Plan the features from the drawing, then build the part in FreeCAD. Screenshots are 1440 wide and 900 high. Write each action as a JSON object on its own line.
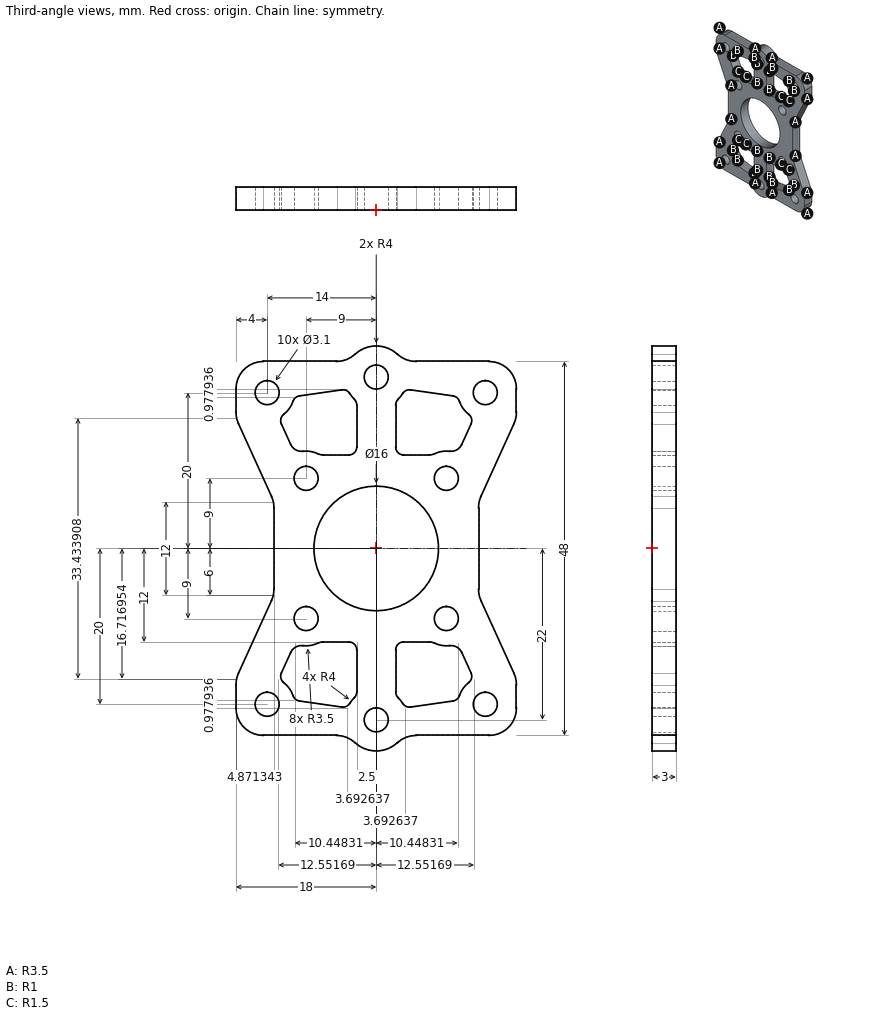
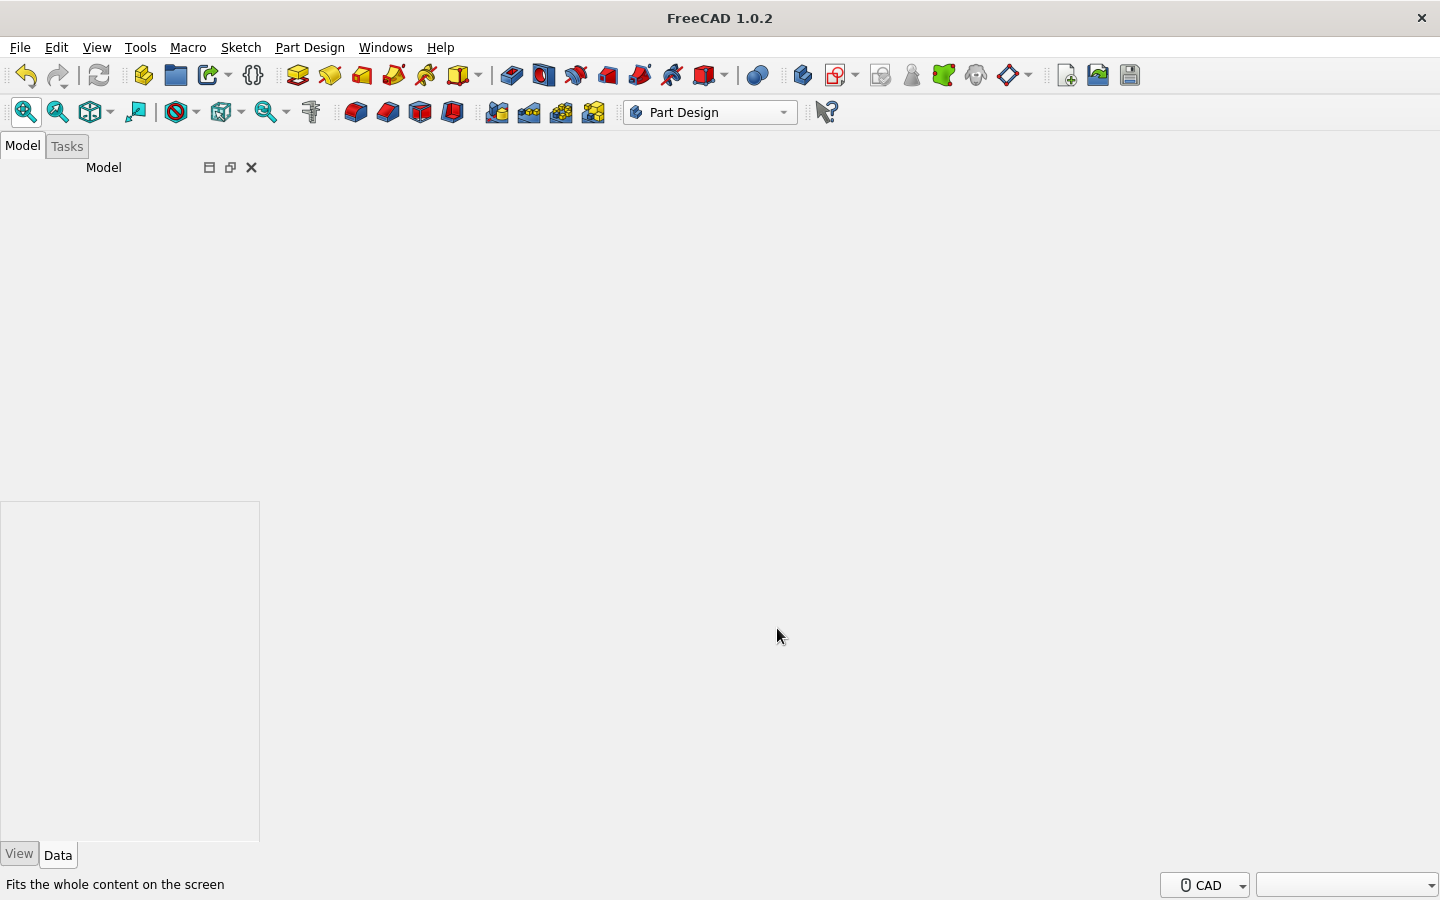
{"action": "left_click", "coordinate": [1066, 76]}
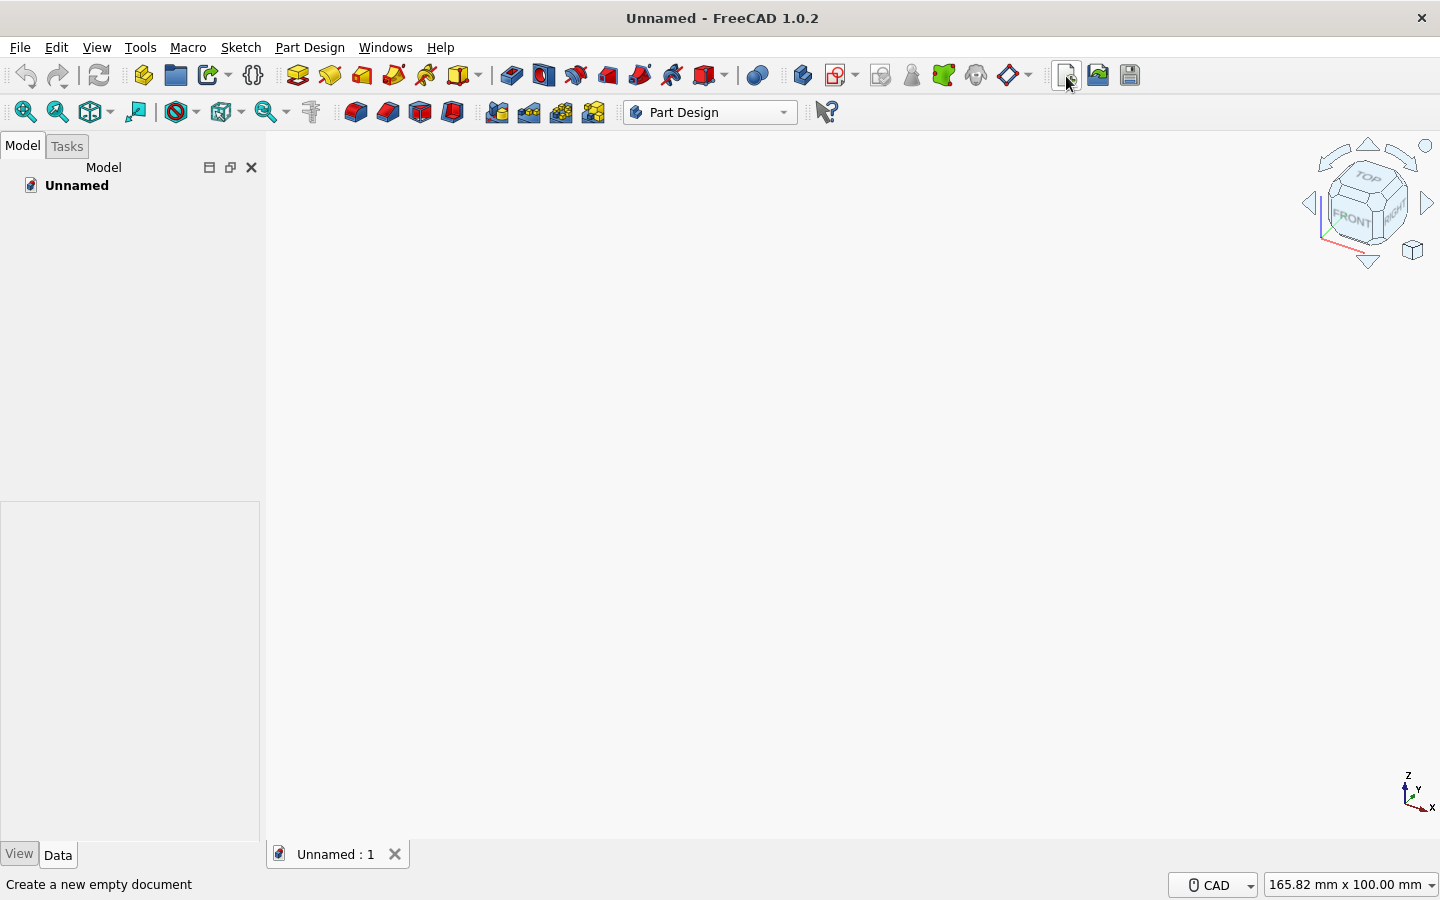
{"action": "left_click", "coordinate": [836, 76]}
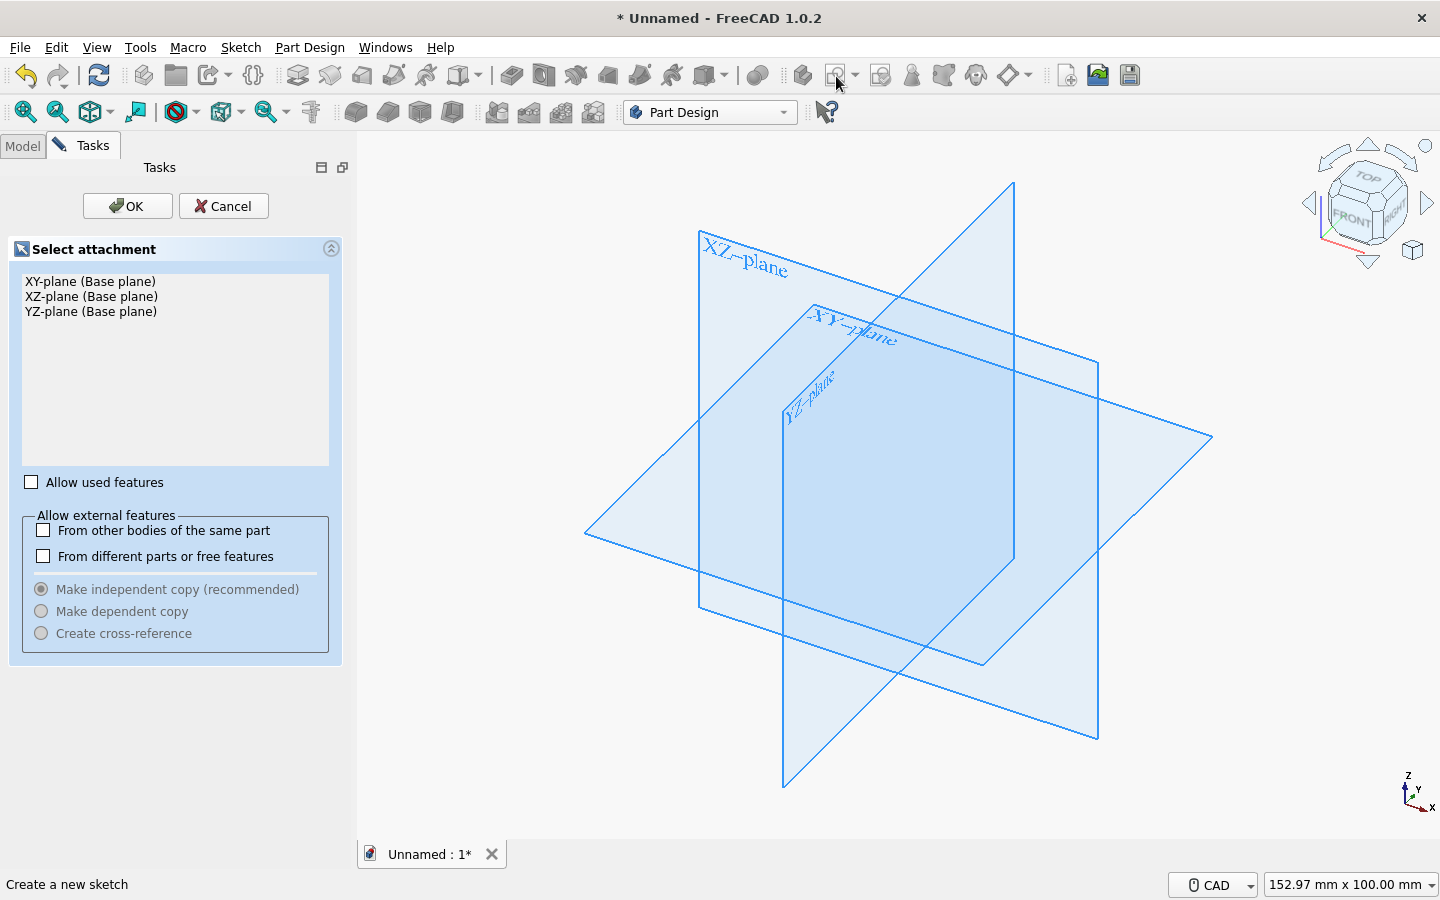
{"action": "left_click", "coordinate": [82, 296]}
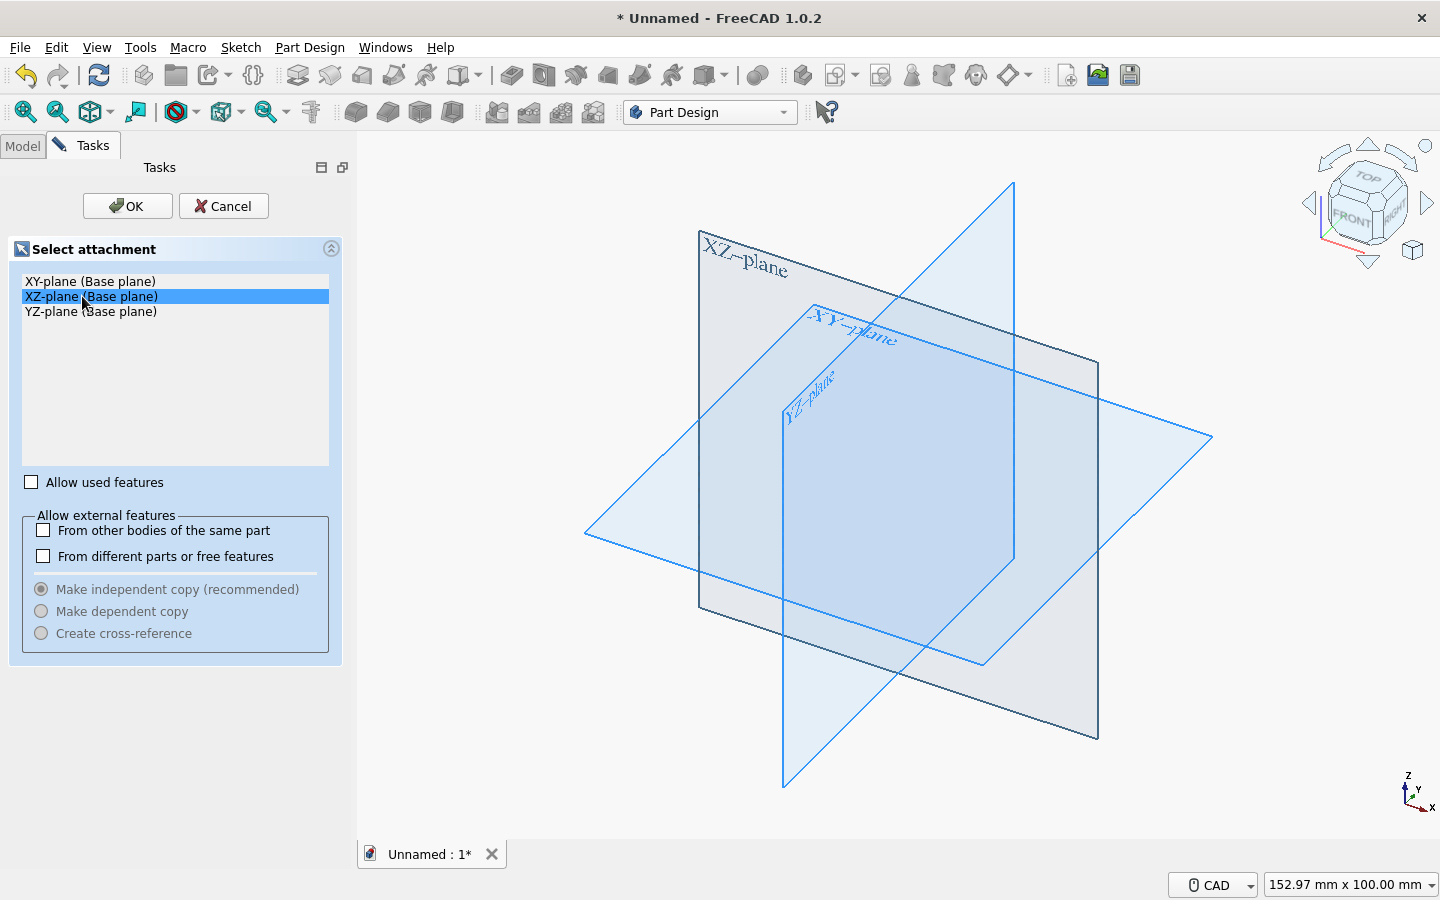
{"action": "left_click", "coordinate": [128, 206]}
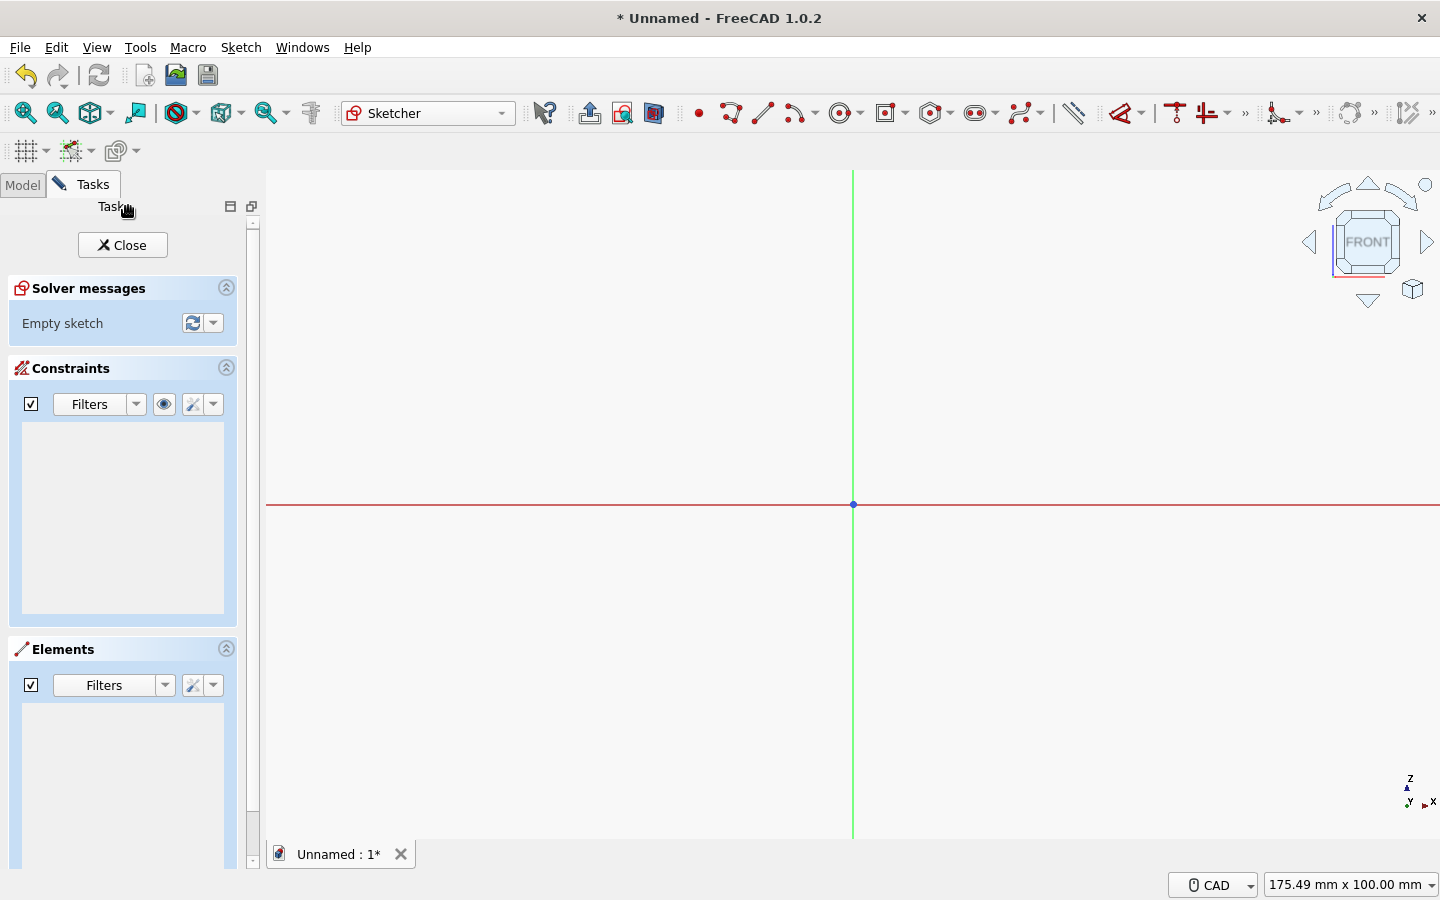
{"action": "left_click", "coordinate": [732, 114]}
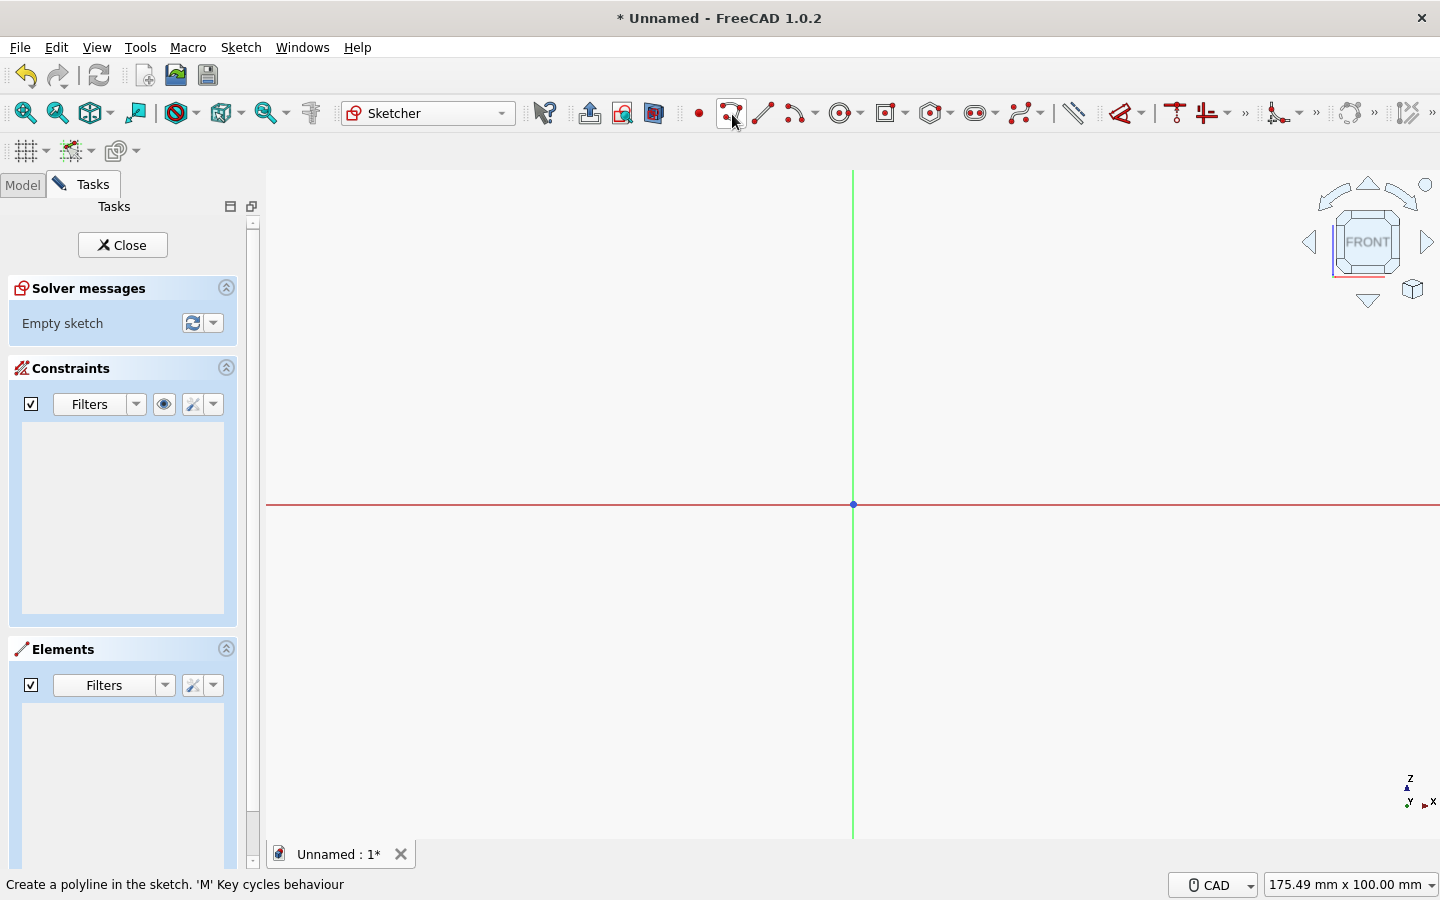
{"action": "left_click", "coordinate": [876, 344]}
{"action": "left_click", "coordinate": [973, 344]}
{"action": "left_click", "coordinate": [973, 665]}
{"action": "left_click", "coordinate": [876, 665]}
{"action": "right_click", "coordinate": [876, 665]}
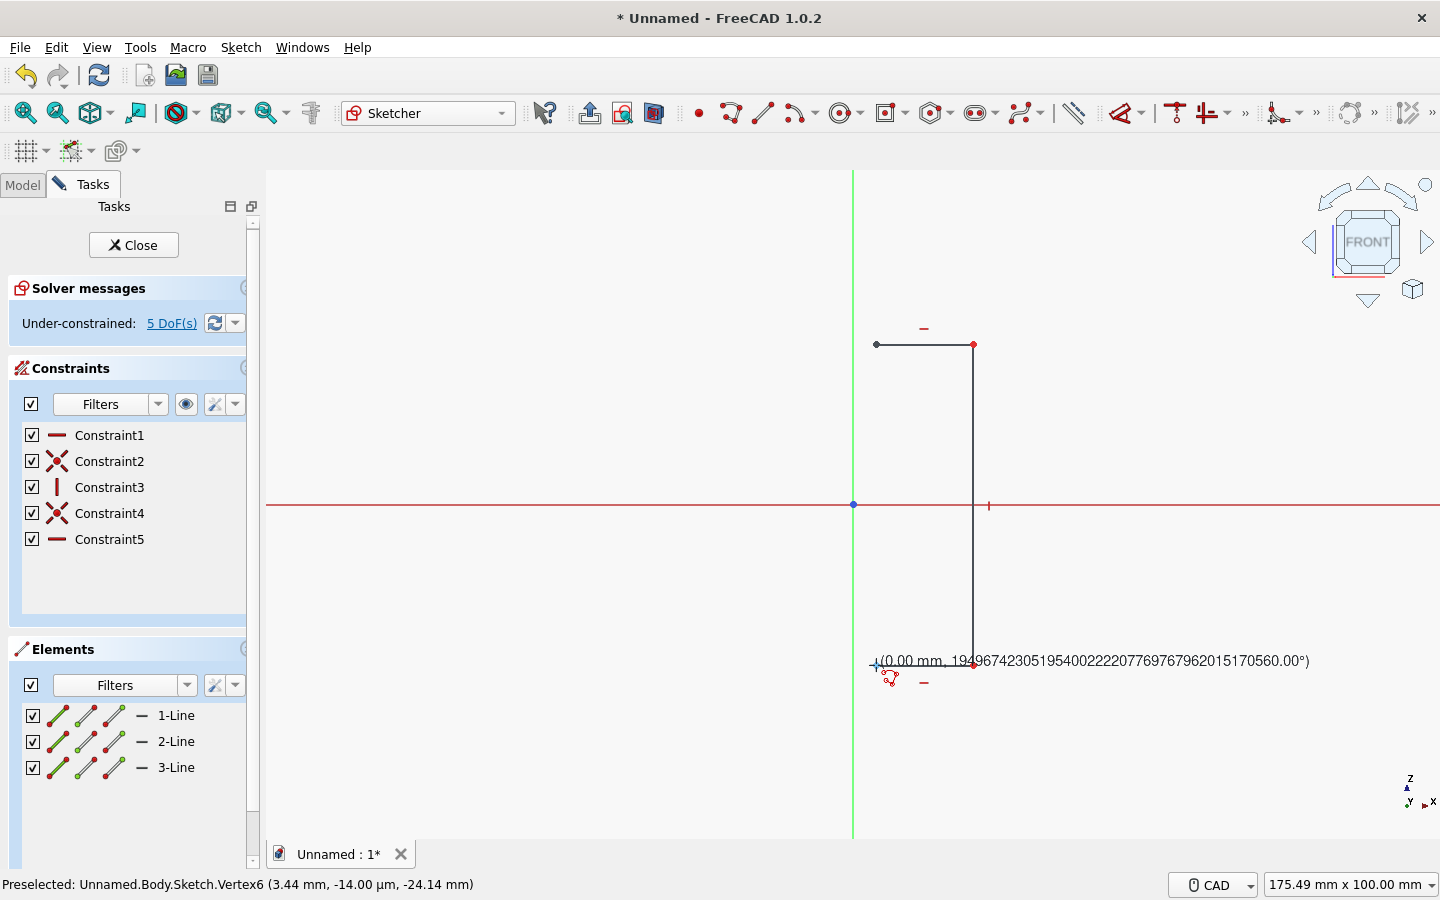
{"action": "left_click", "coordinate": [830, 665]}
{"action": "left_click", "coordinate": [733, 665]}
{"action": "left_click", "coordinate": [733, 344]}
{"action": "left_click", "coordinate": [830, 344]}
{"action": "right_click", "coordinate": [830, 344]}